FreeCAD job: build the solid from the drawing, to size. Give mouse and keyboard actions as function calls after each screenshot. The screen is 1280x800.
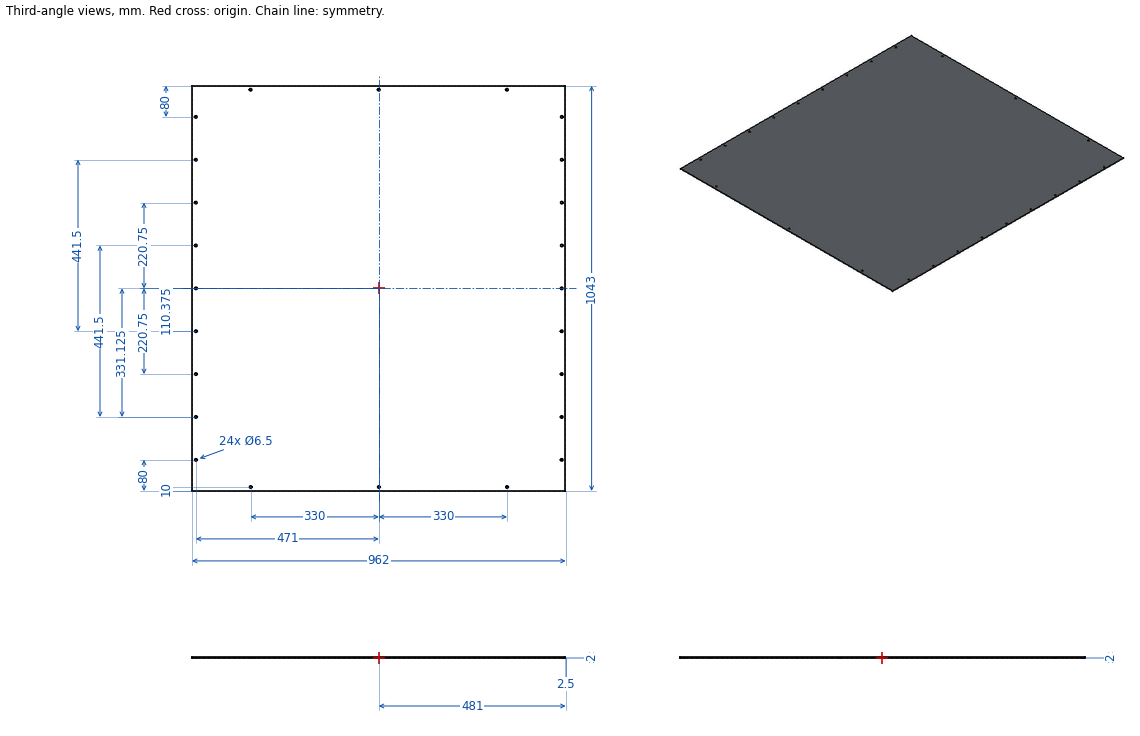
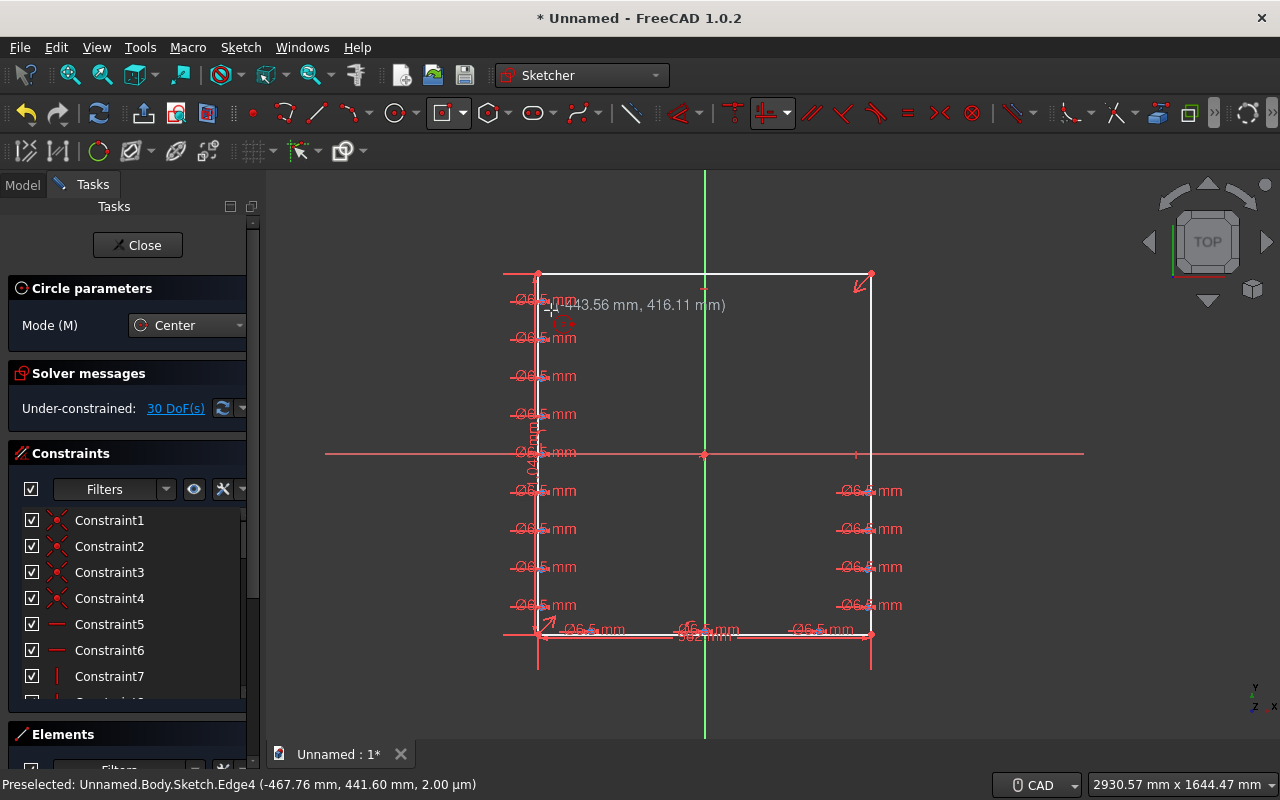
scroll(591, 277, up, 16)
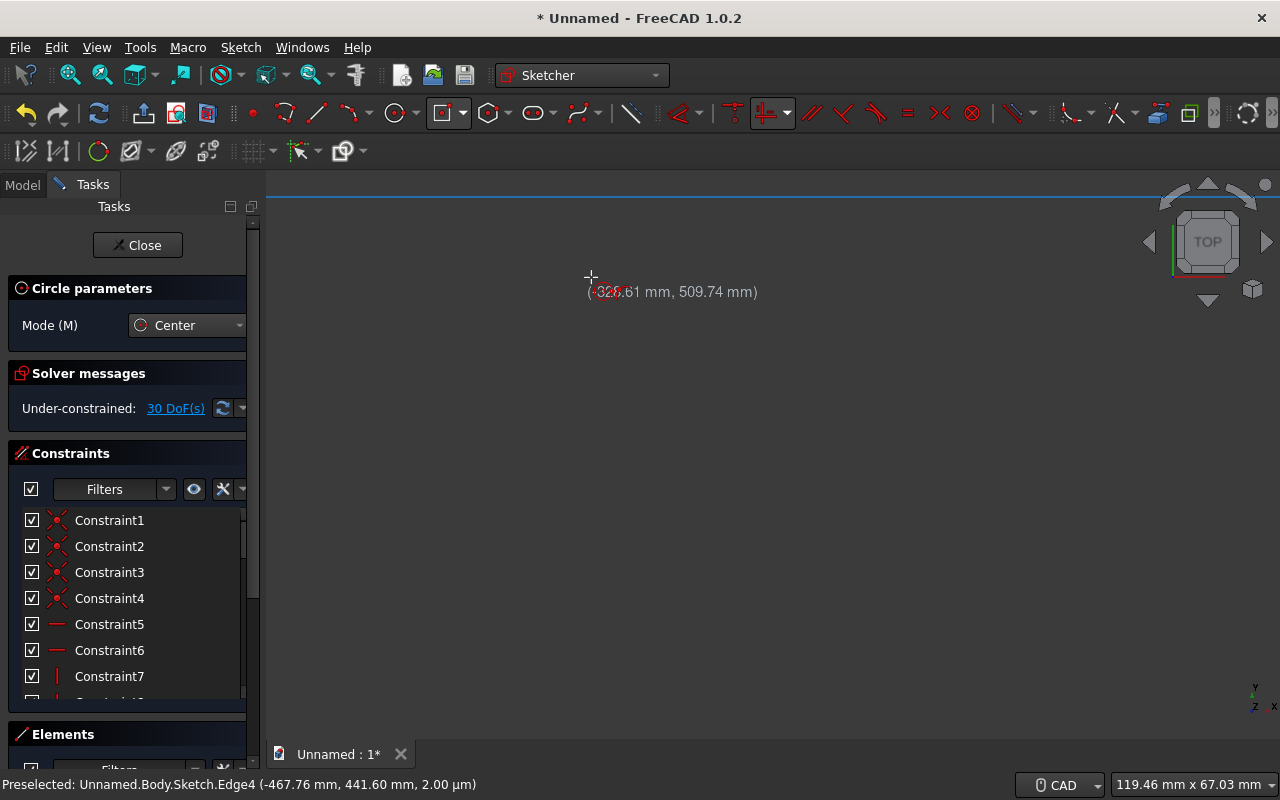
scroll(565, 236, down, 15)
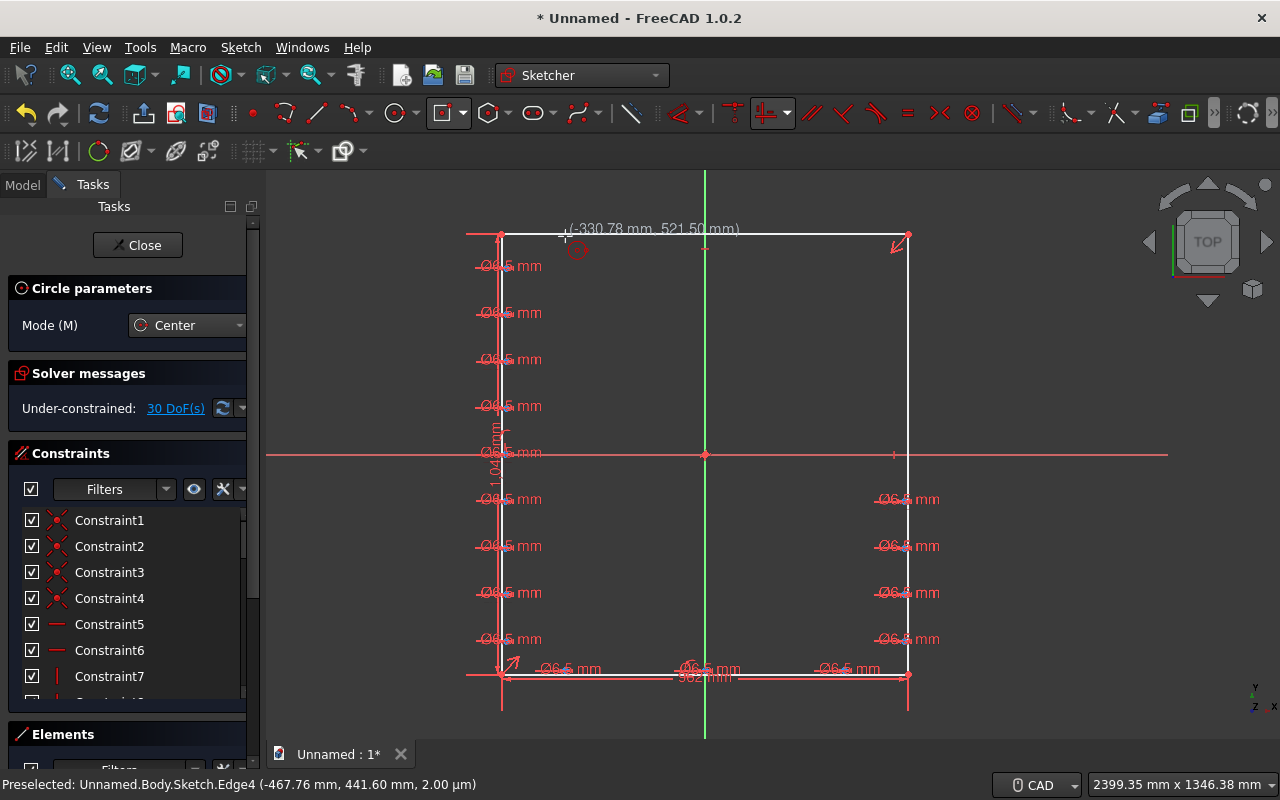
scroll(566, 238, up, 7)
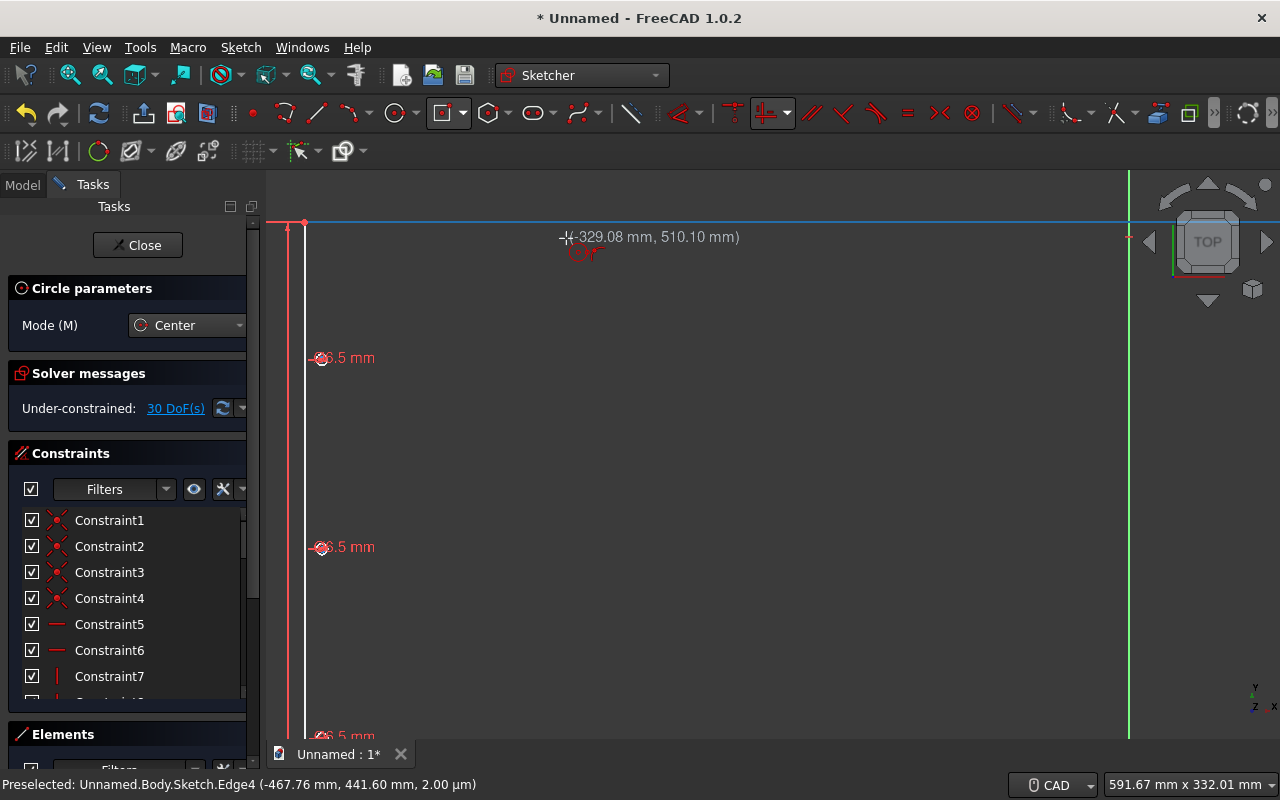
click(564, 239)
move(567, 243)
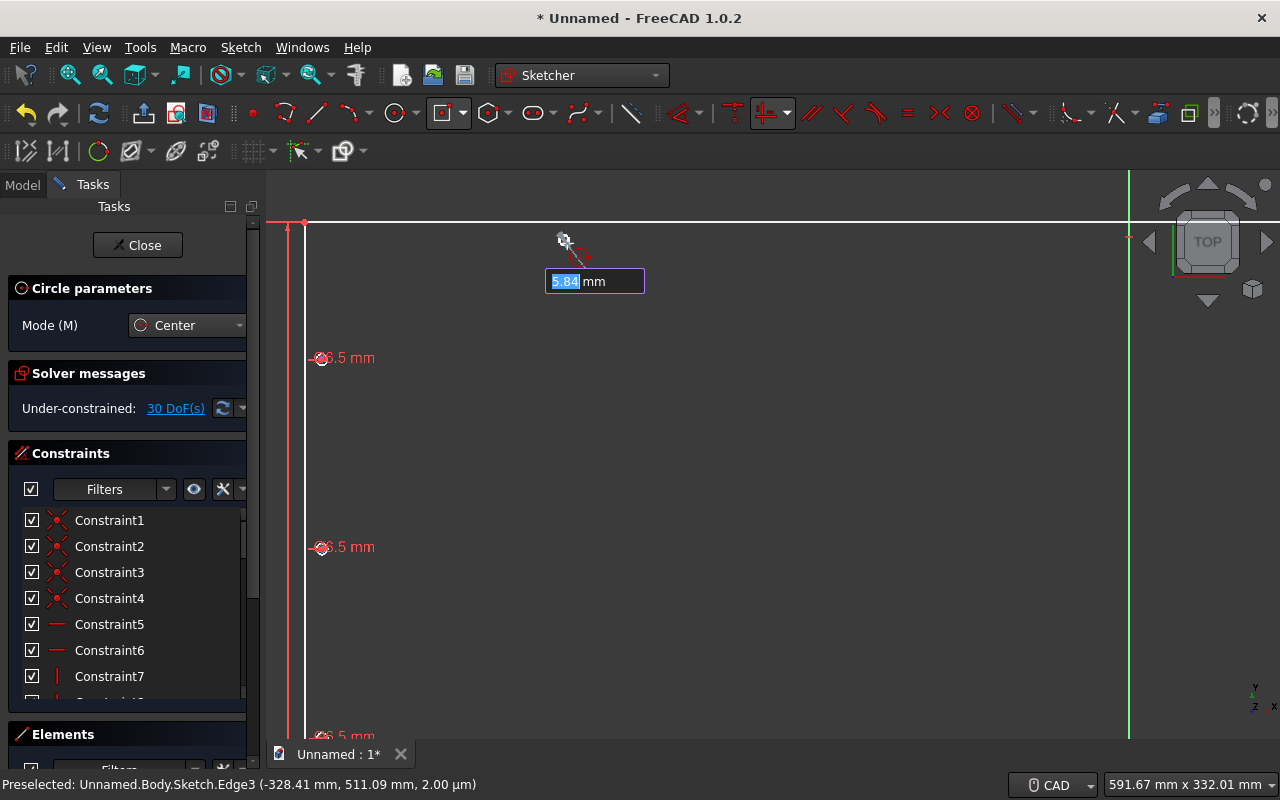
text(6.5)
key(Return)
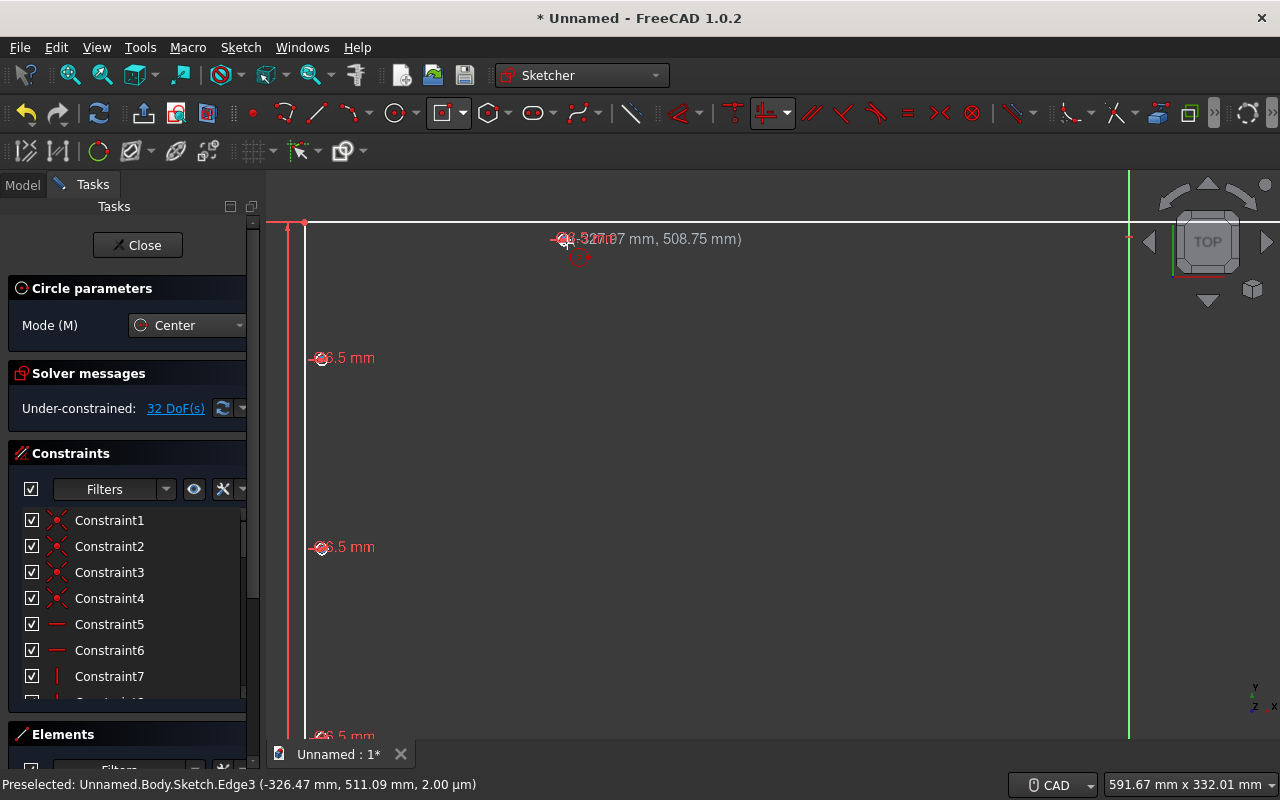
scroll(597, 287, down, 8)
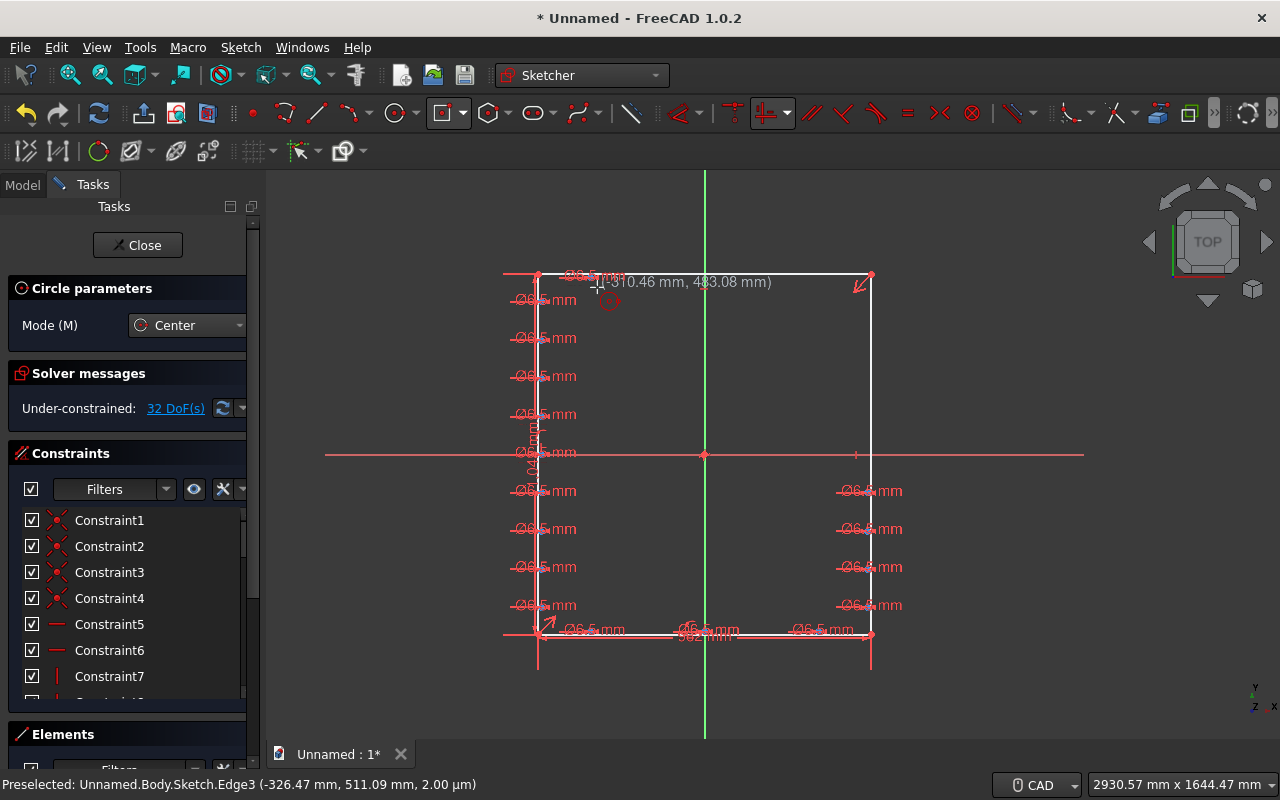
scroll(868, 455, up, 16)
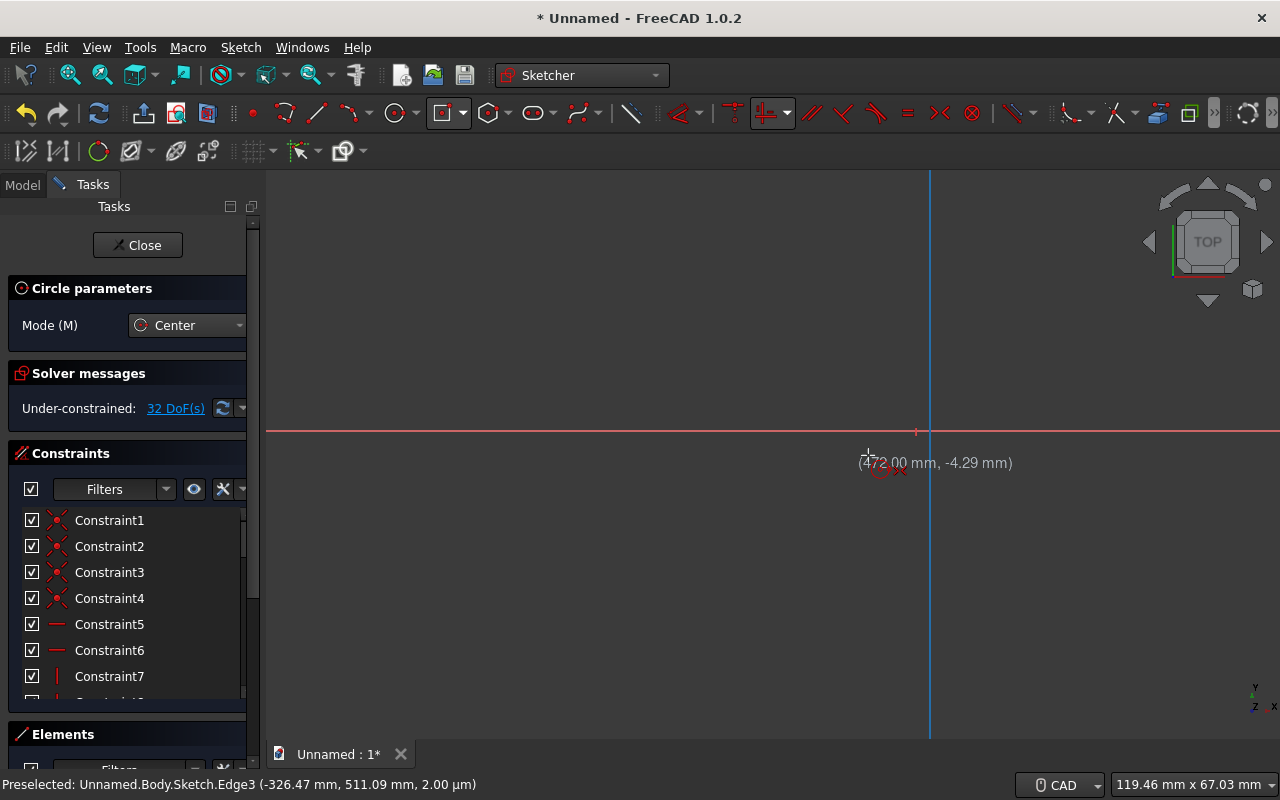
scroll(907, 456, down, 15)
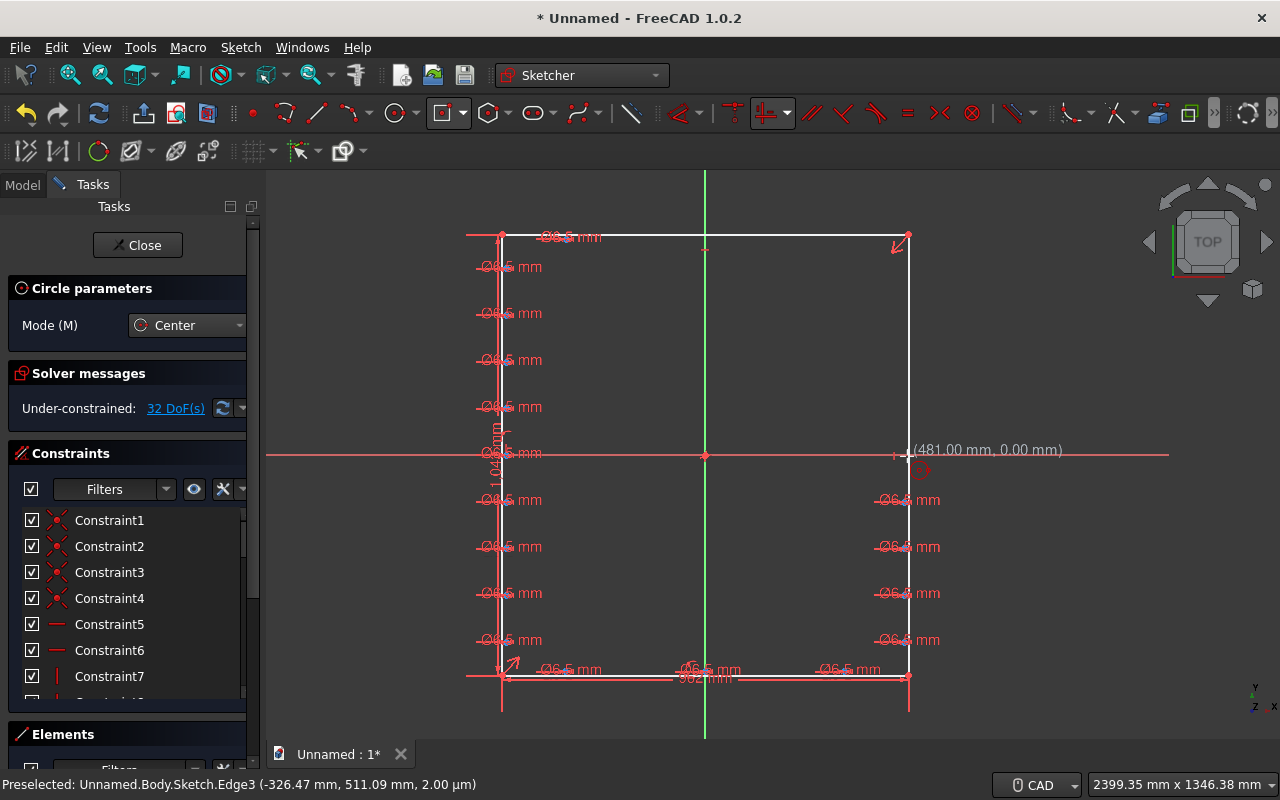
scroll(905, 455, up, 7)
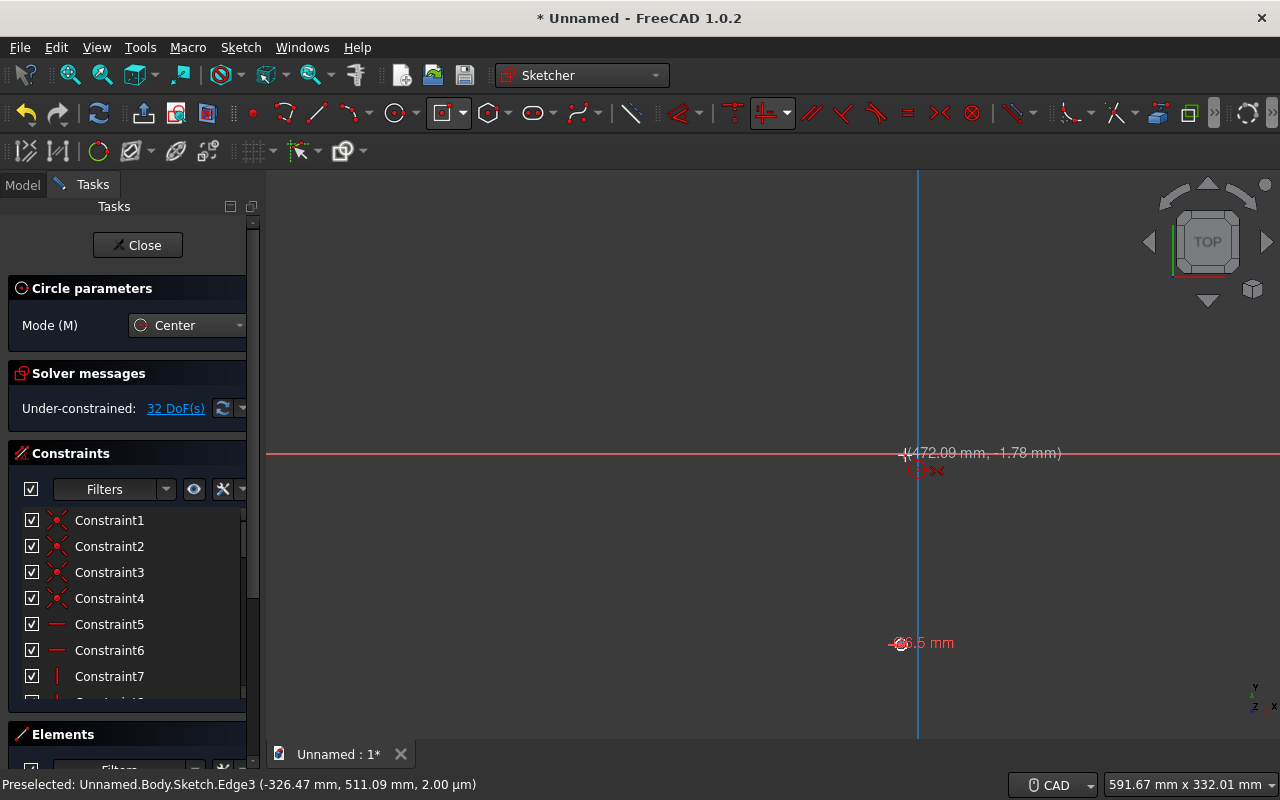
click(901, 454)